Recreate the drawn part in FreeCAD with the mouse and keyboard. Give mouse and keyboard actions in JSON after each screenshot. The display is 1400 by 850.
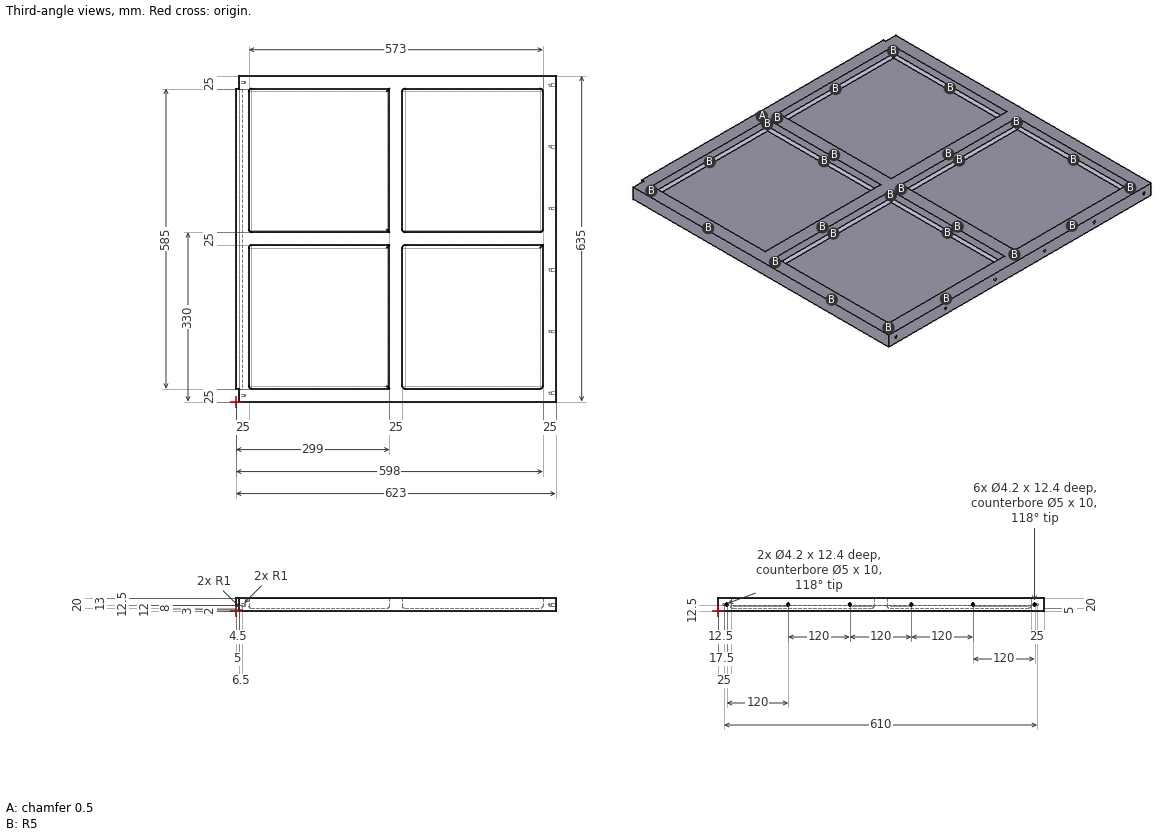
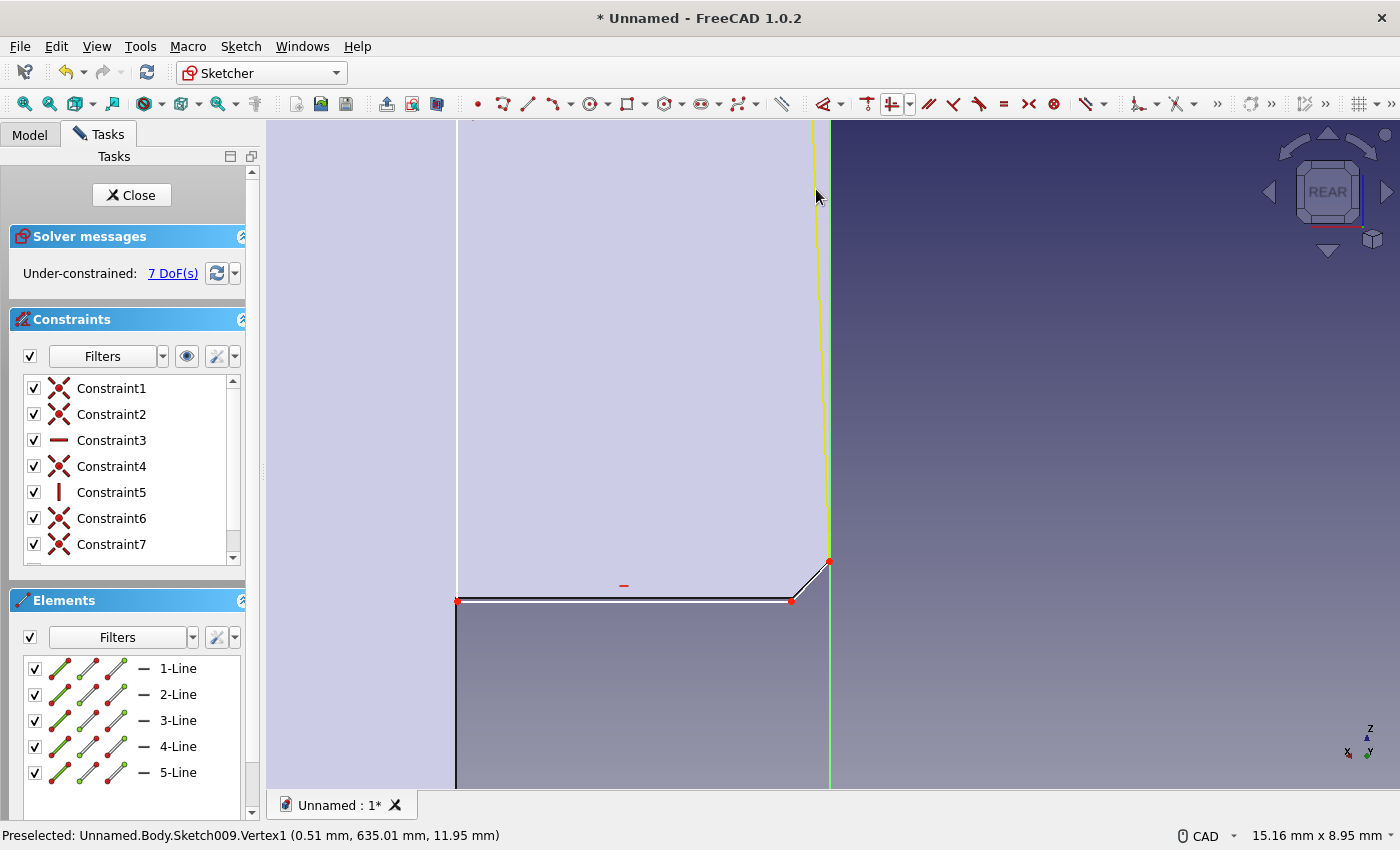
{"action": "left_click", "coordinate": [815, 189]}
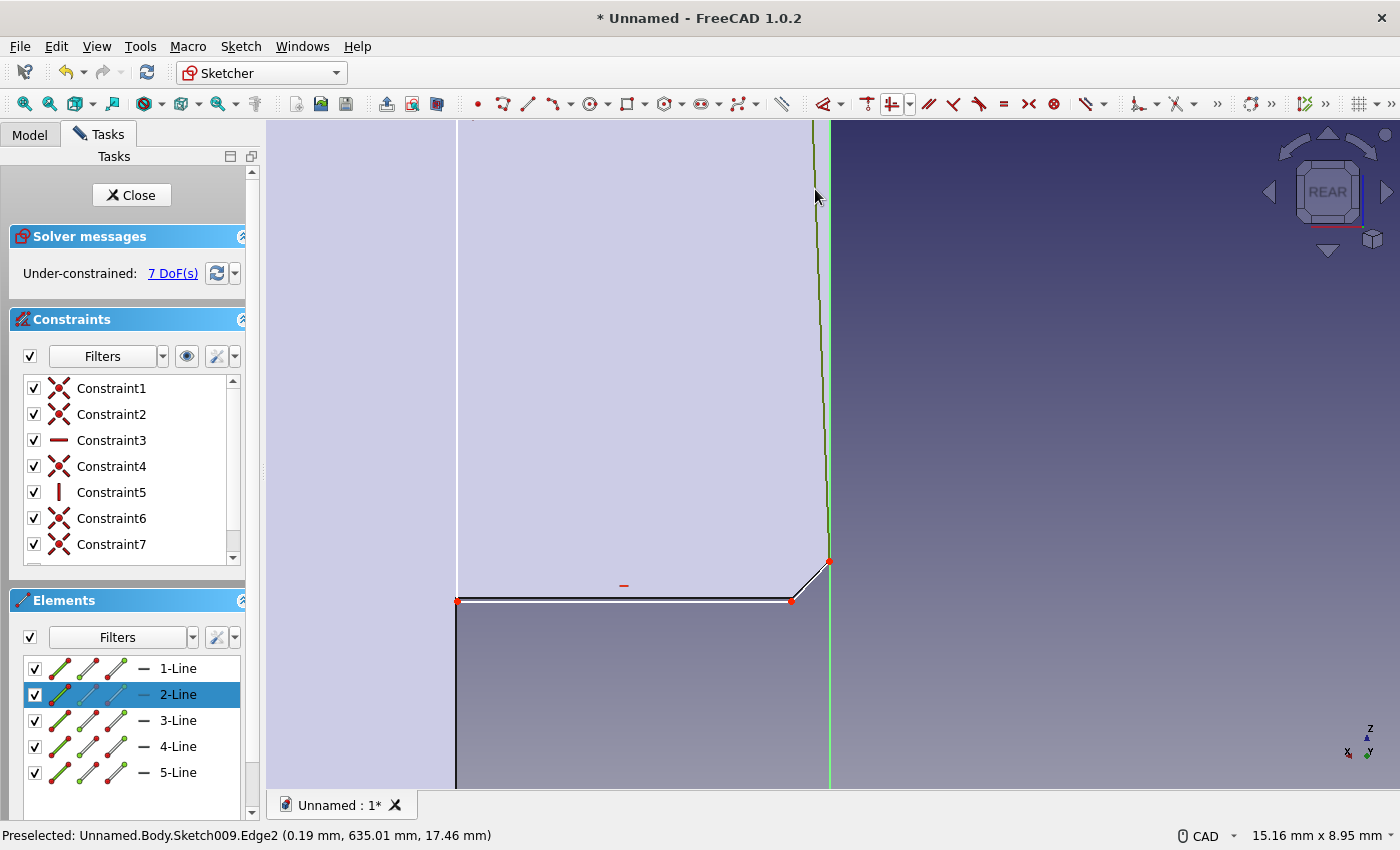
{"action": "left_click", "coordinate": [910, 104]}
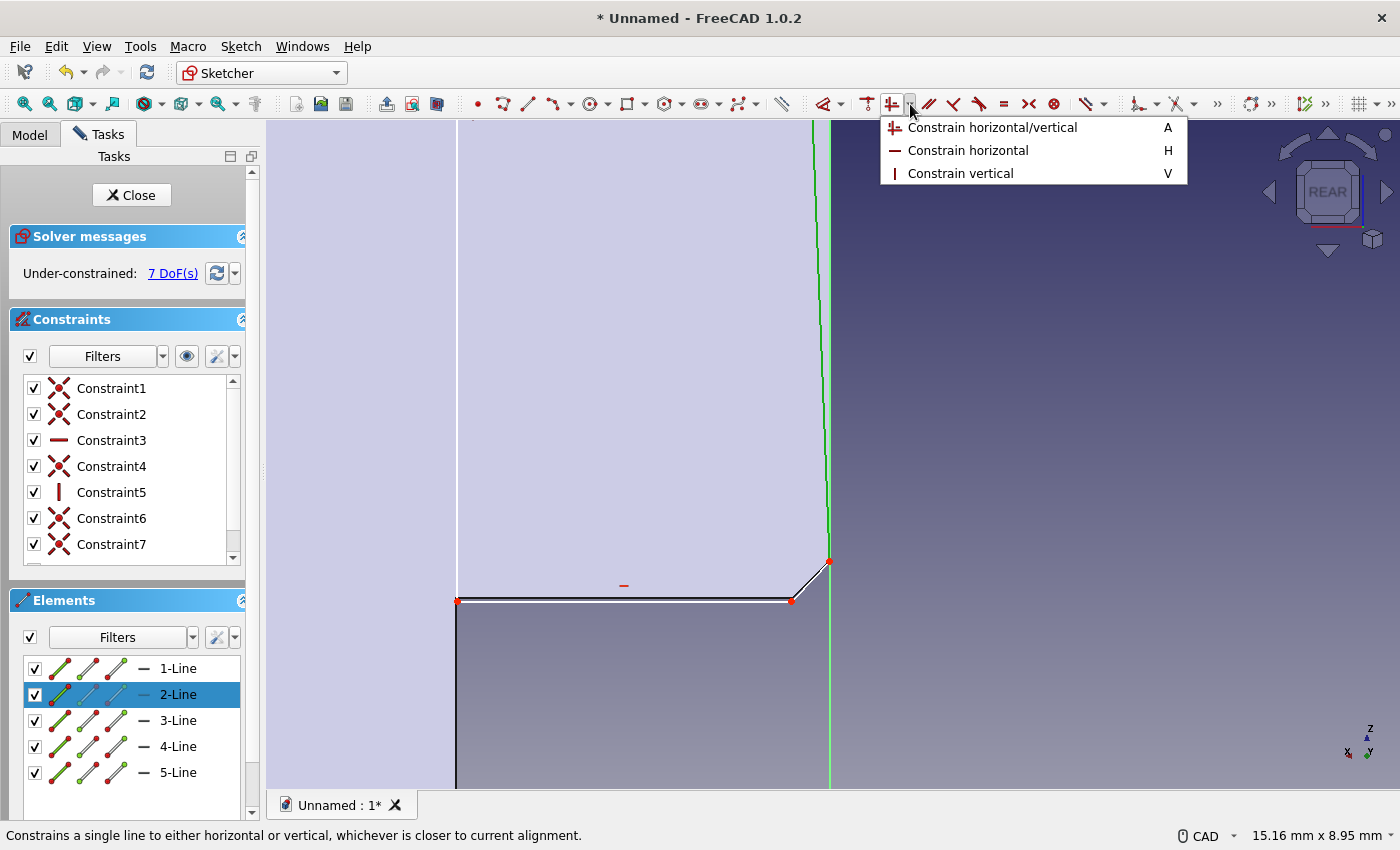
{"action": "left_click", "coordinate": [1034, 174]}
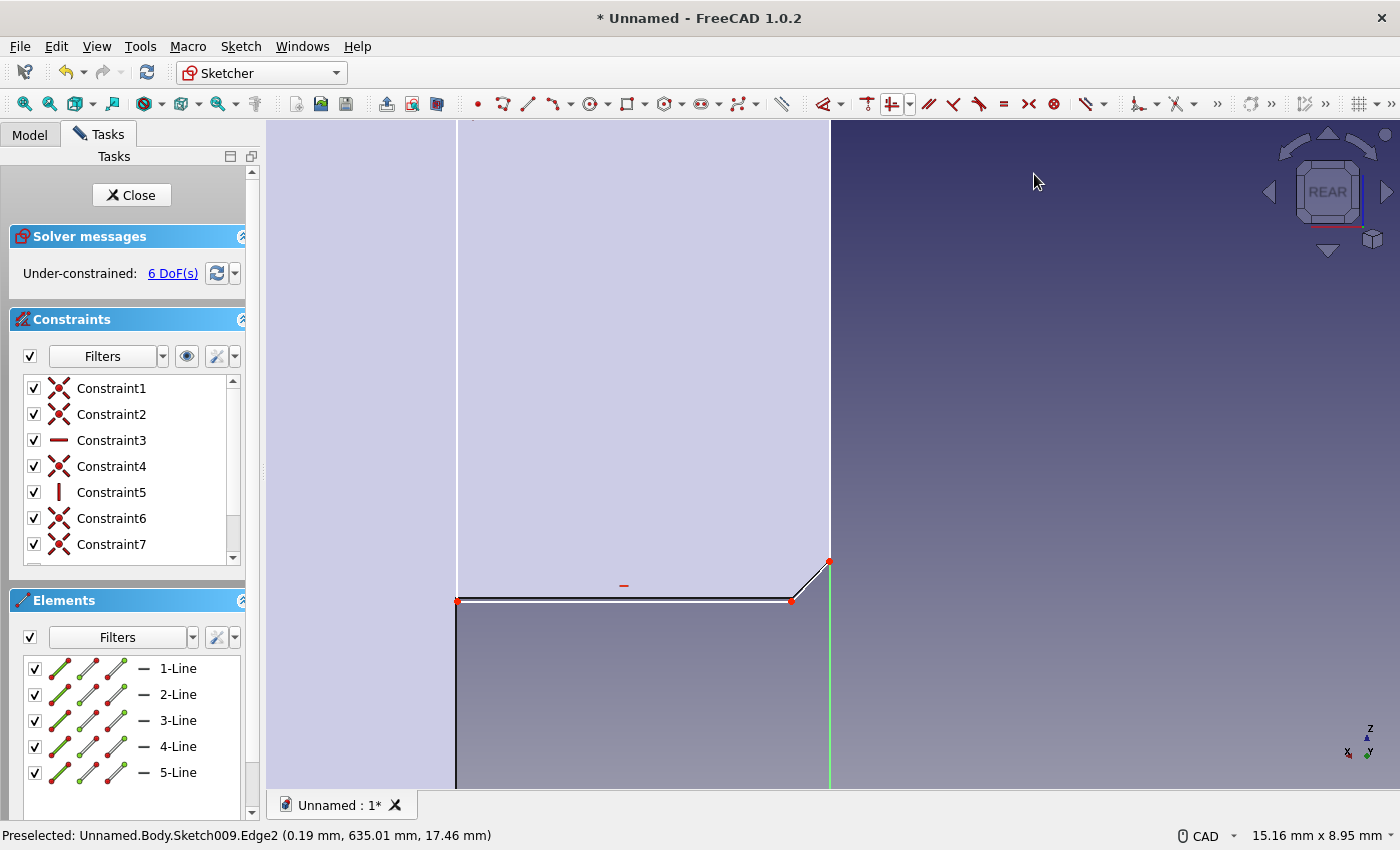
{"action": "scroll", "coordinate": [804, 420], "scroll_direction": "down", "scroll_amount": 7}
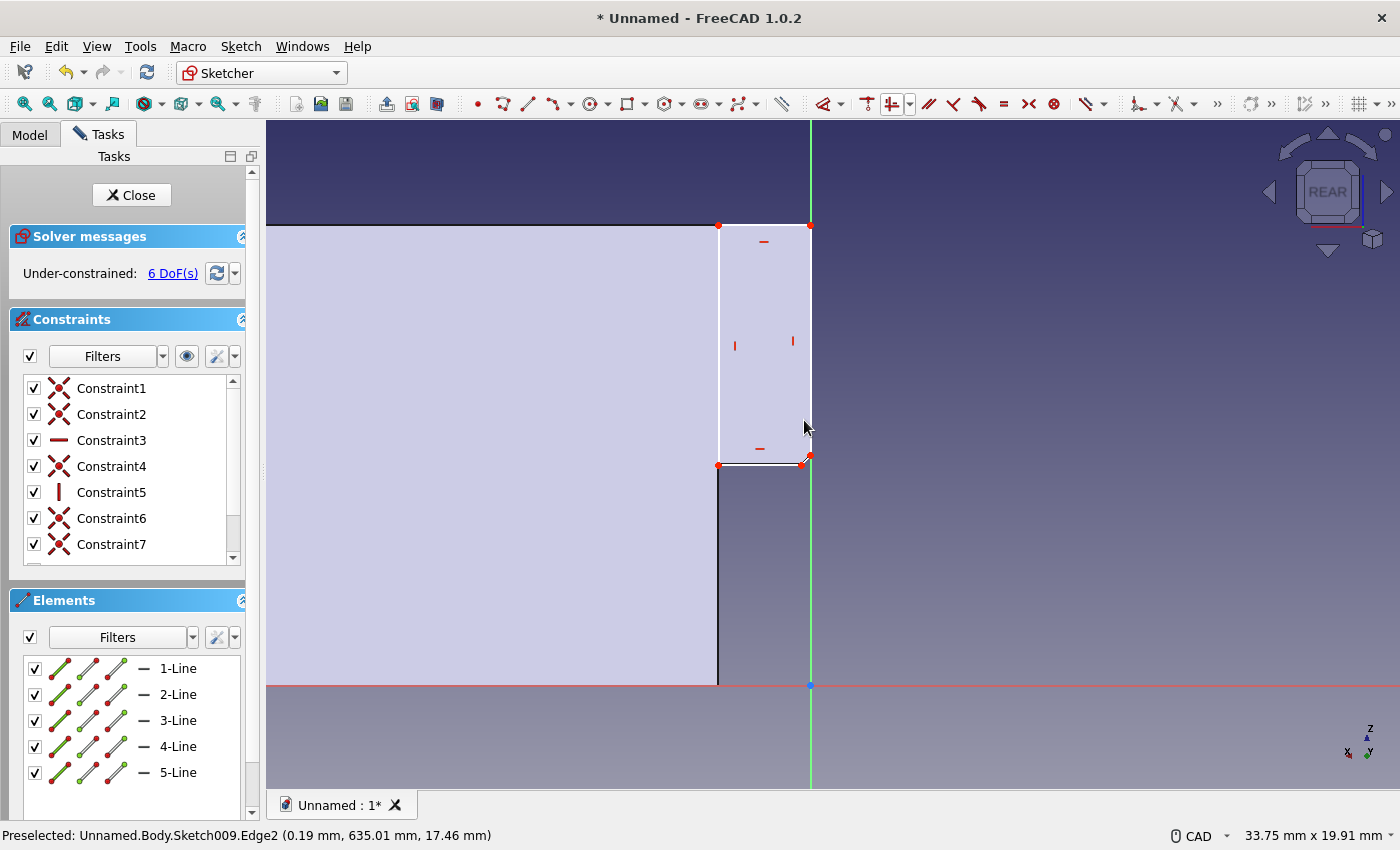
{"action": "left_click", "coordinate": [811, 455]}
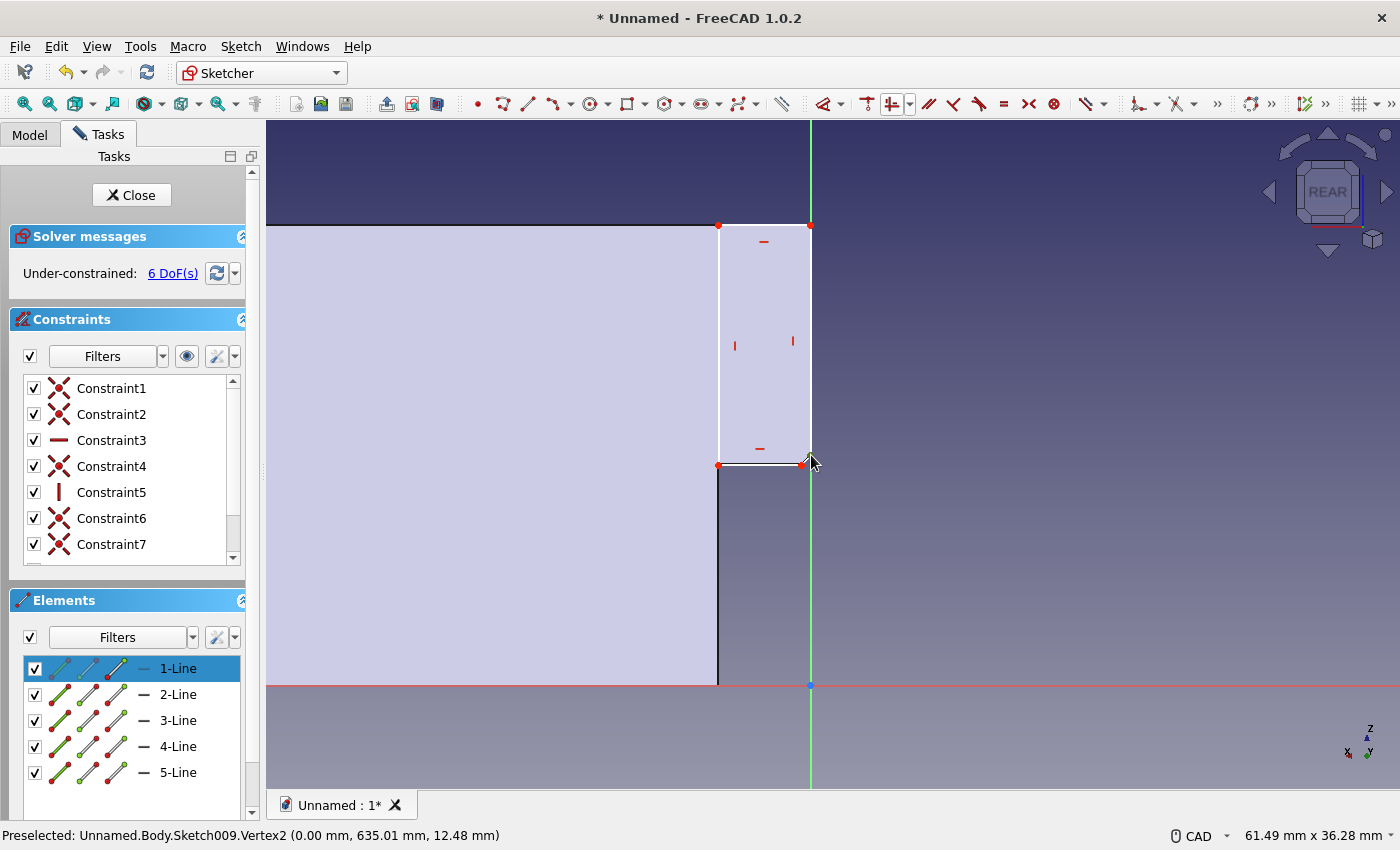
{"action": "left_click", "coordinate": [811, 717]}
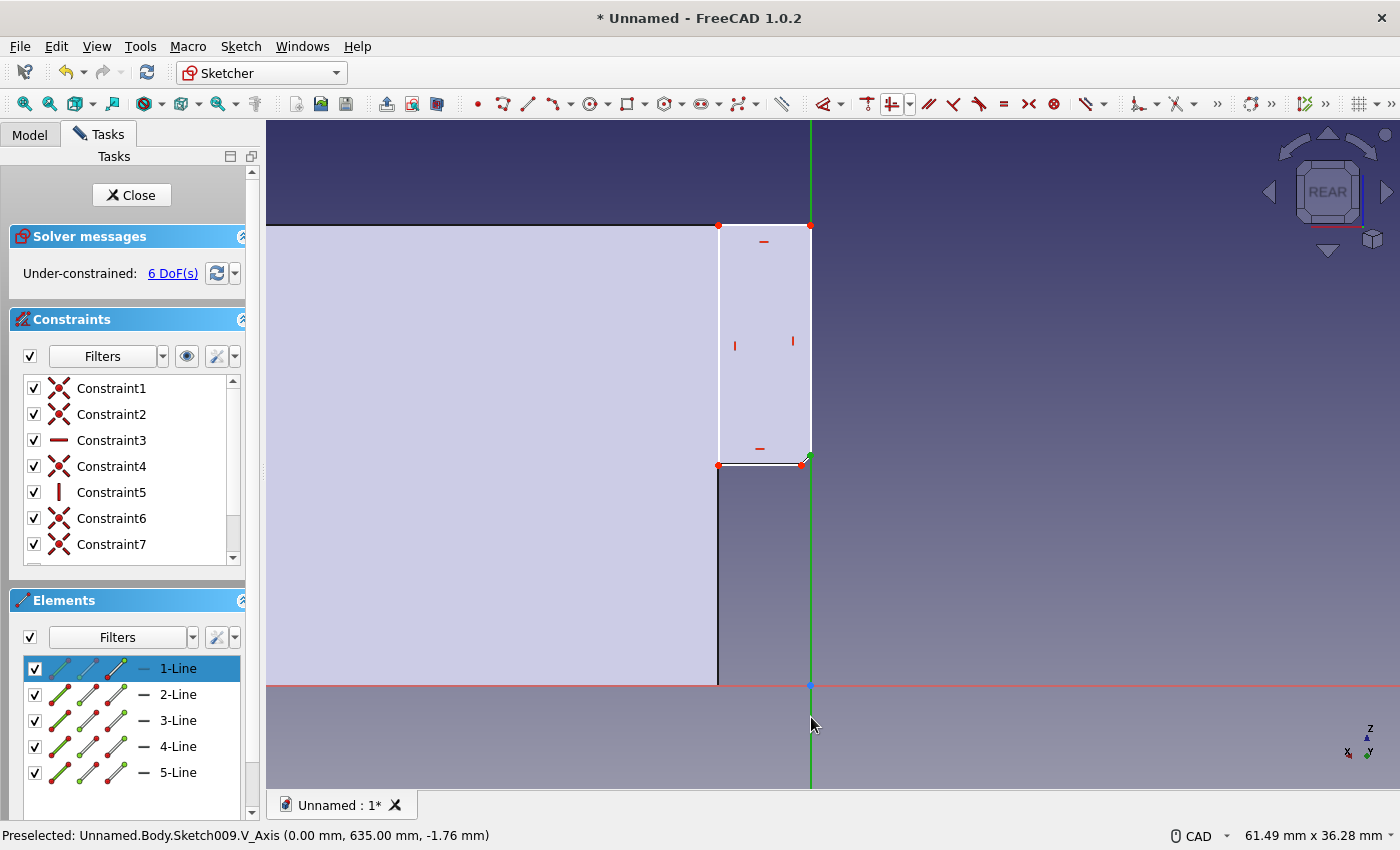
{"action": "left_click", "coordinate": [867, 104]}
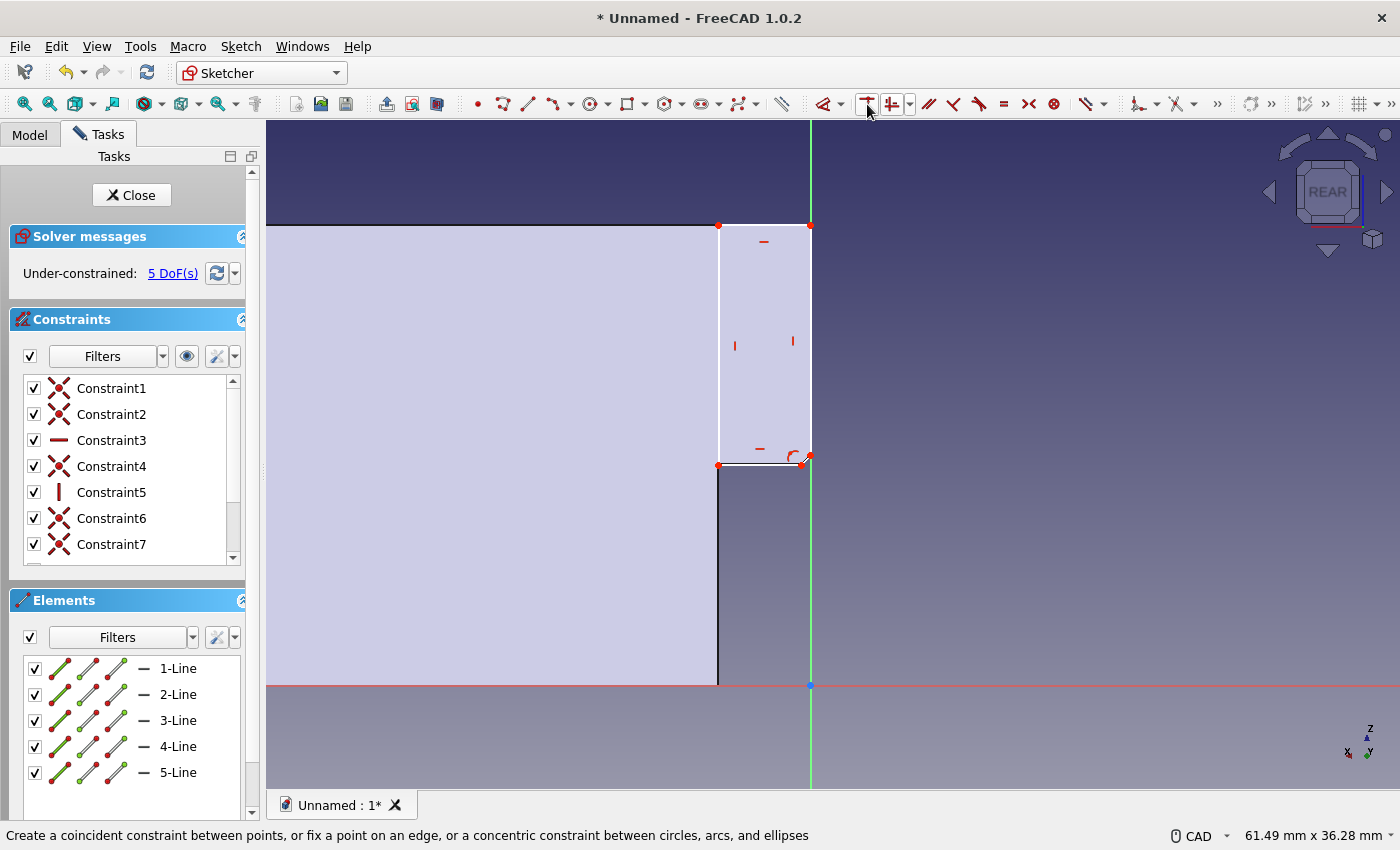
{"action": "left_click", "coordinate": [822, 104]}